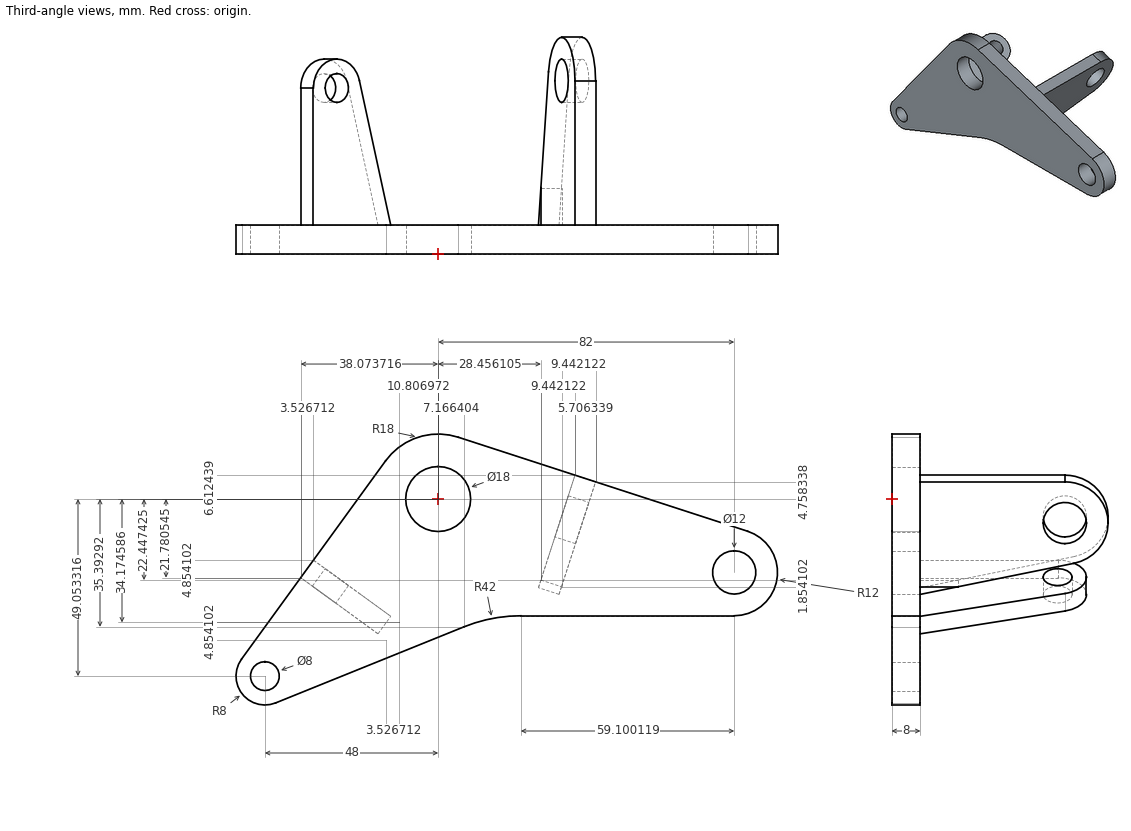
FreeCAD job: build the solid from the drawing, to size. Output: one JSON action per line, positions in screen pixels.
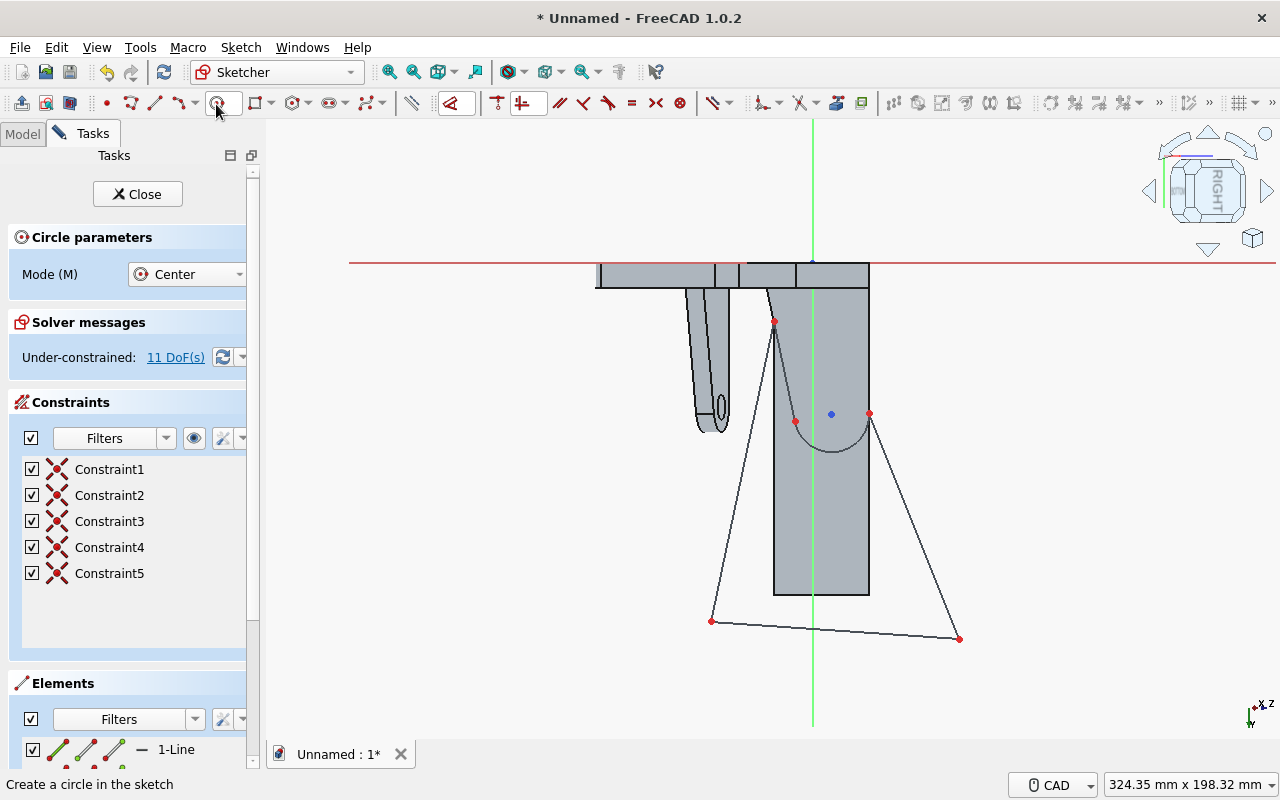
{"action": "left_click", "coordinate": [832, 413]}
{"action": "mouse_move", "coordinate": [845, 400]}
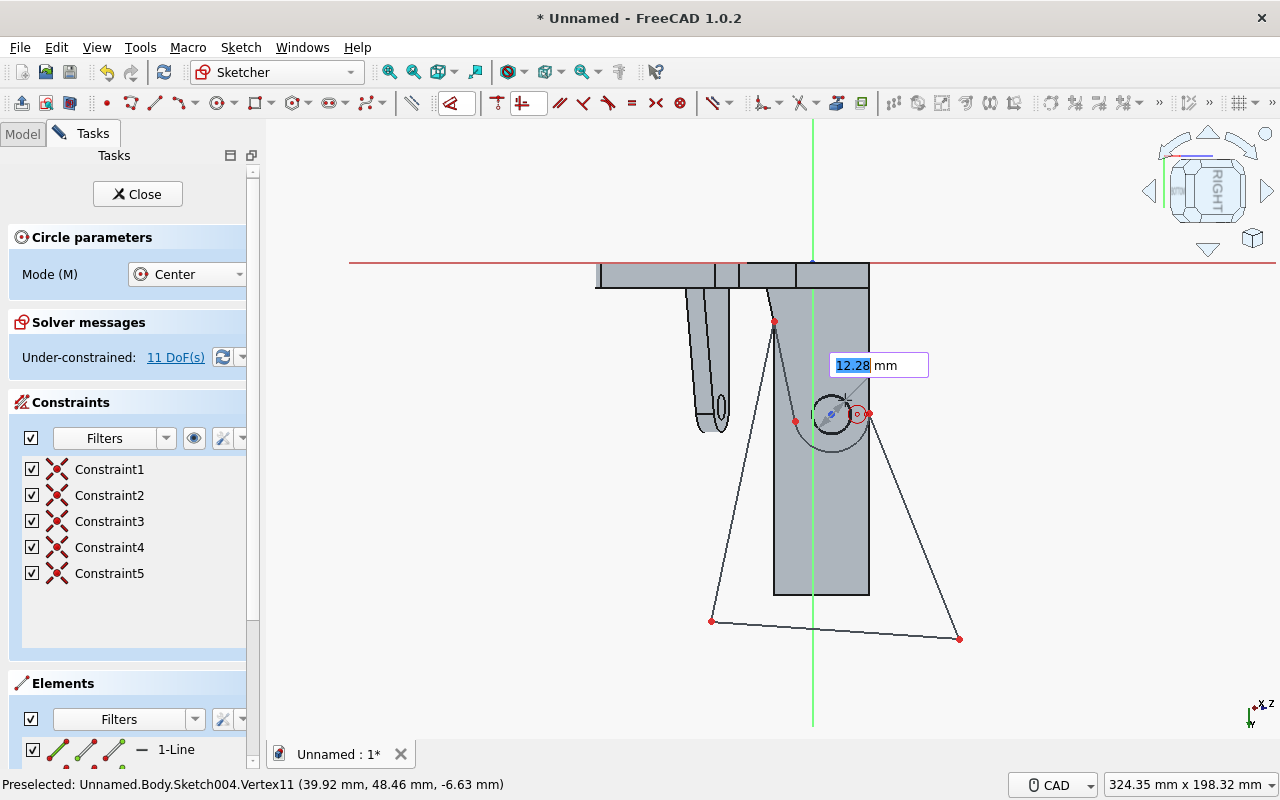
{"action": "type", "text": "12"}
{"action": "key", "text": "Return"}
{"action": "key", "text": "Escape"}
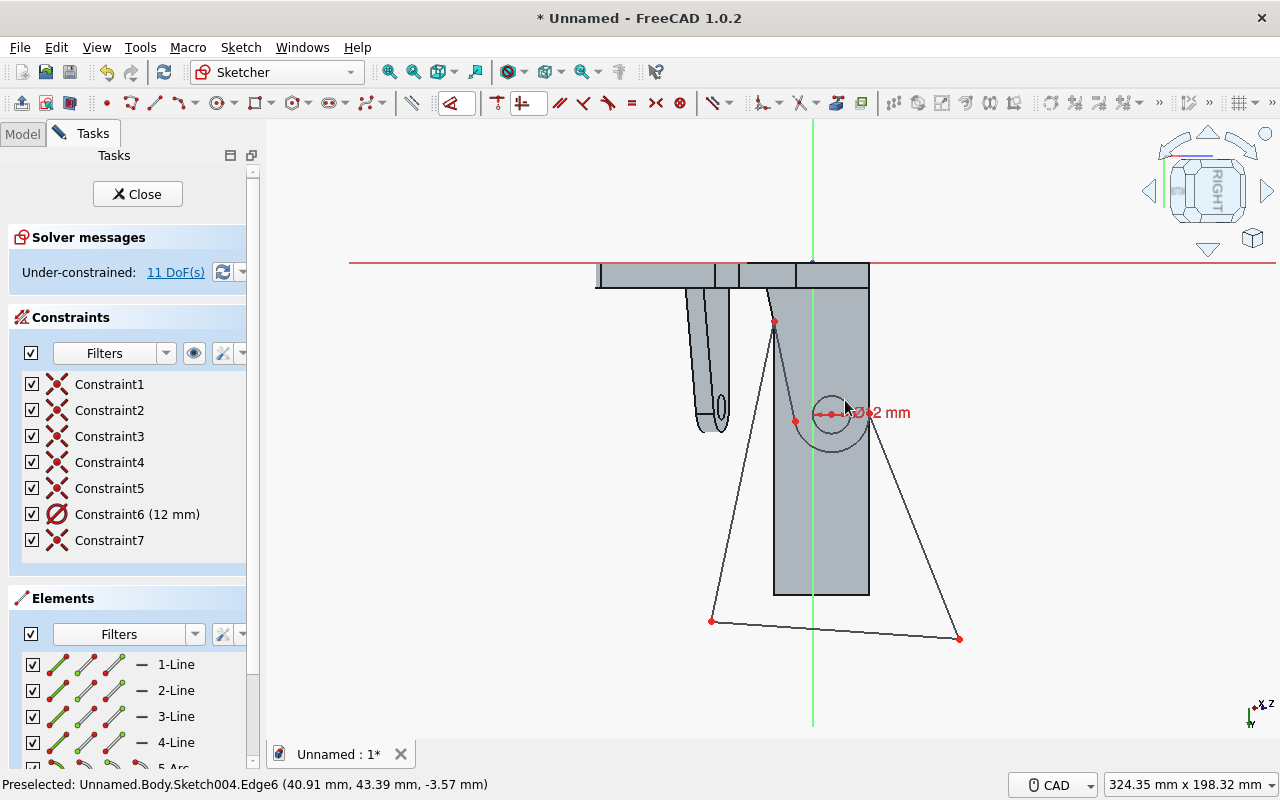
{"action": "left_click", "coordinate": [789, 392]}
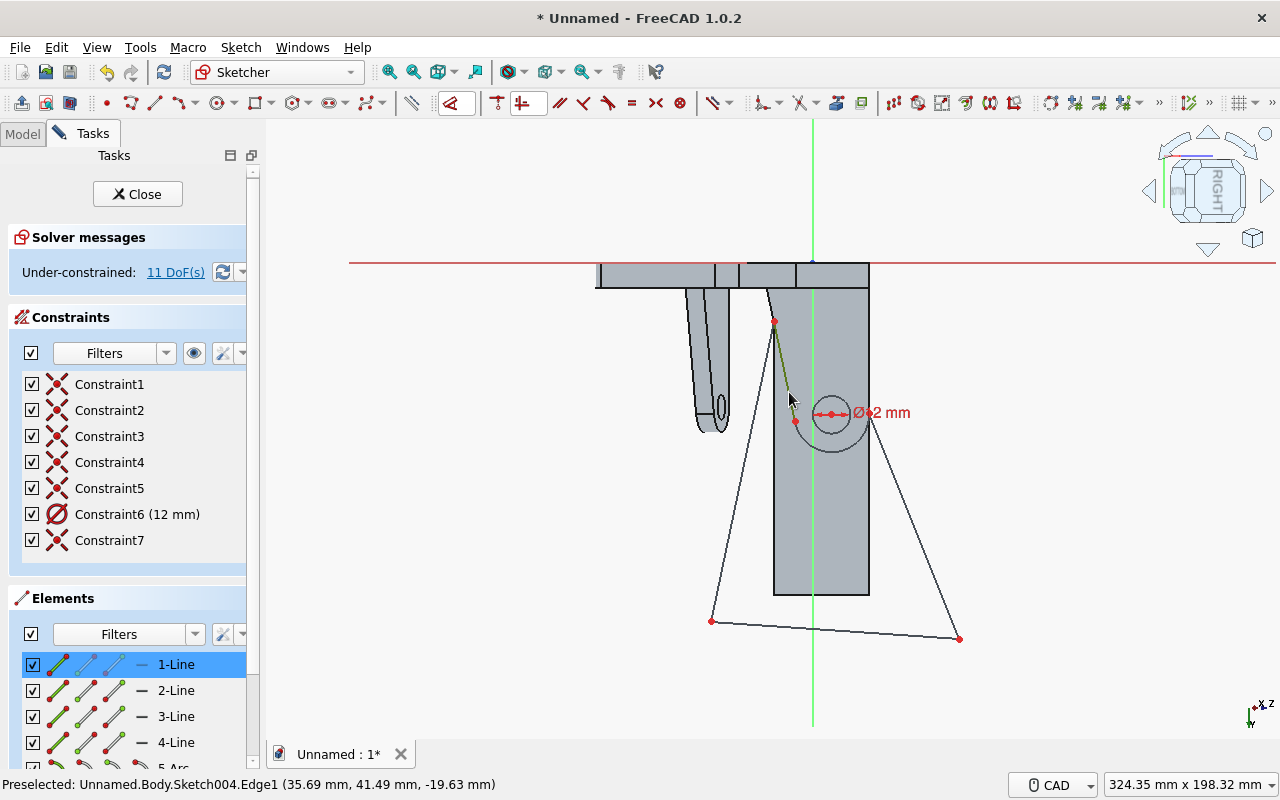
{"action": "left_click", "coordinate": [814, 448]}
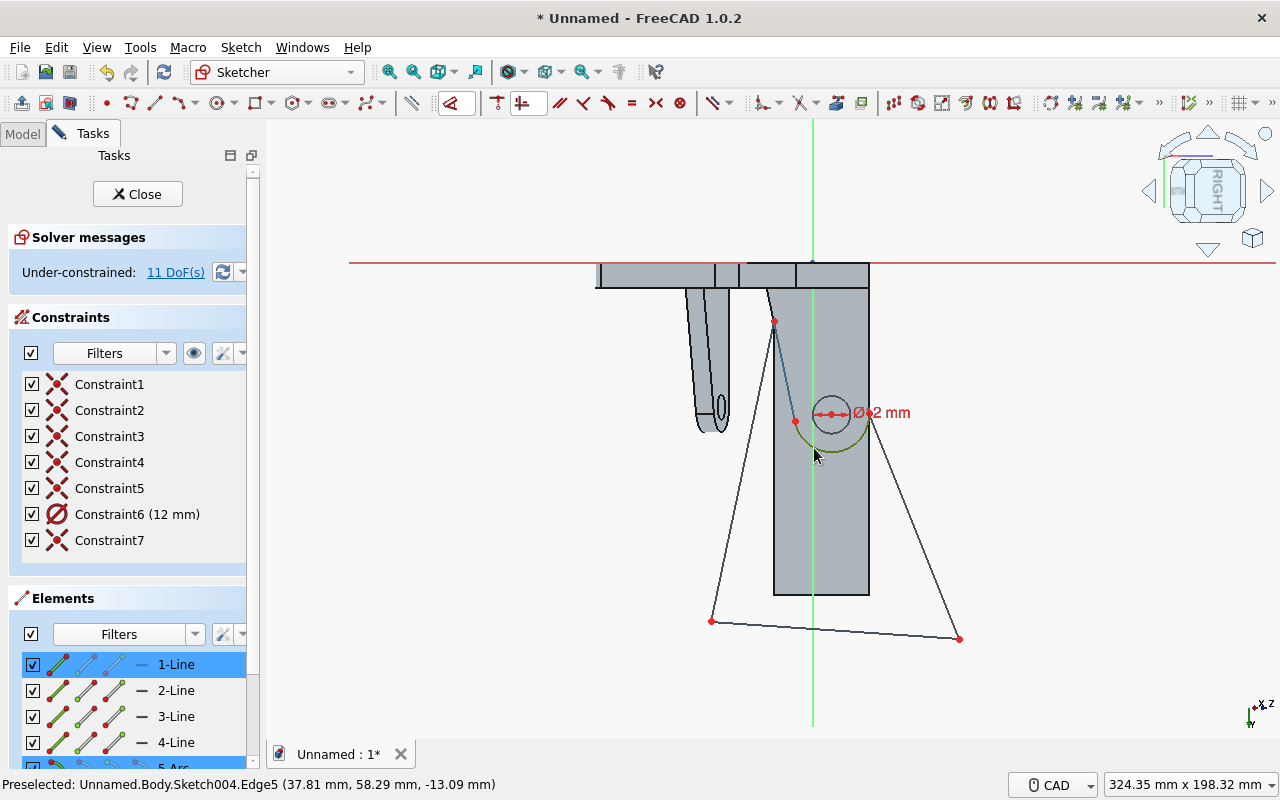
{"action": "key", "text": "t"}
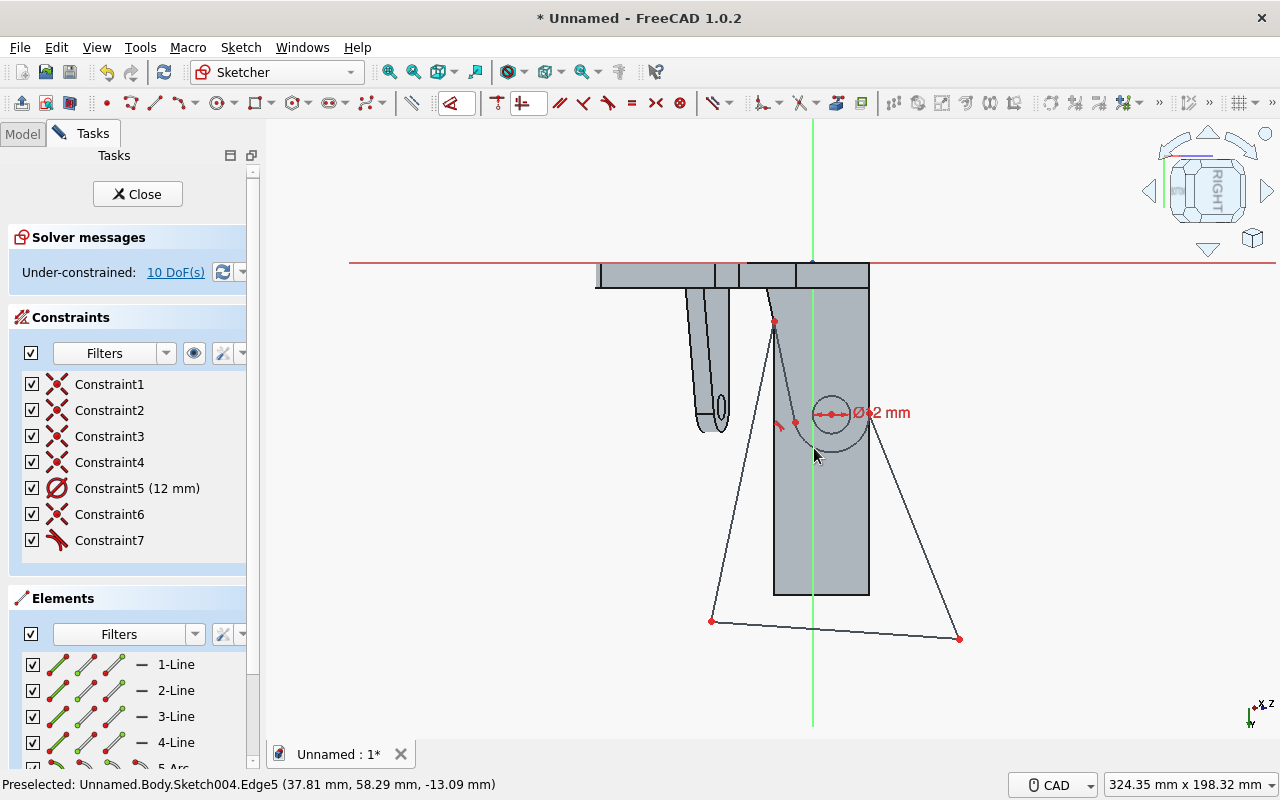
{"action": "left_click", "coordinate": [814, 448]}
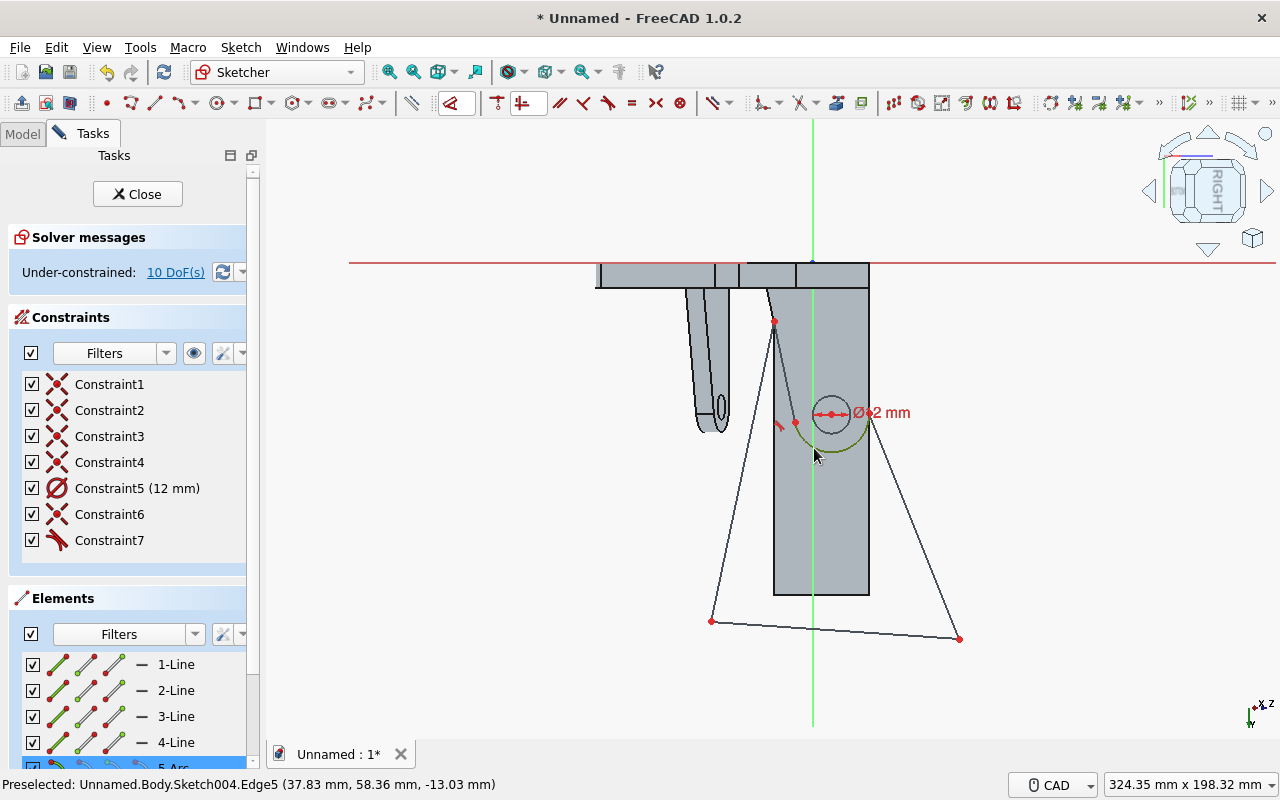
{"action": "left_click", "coordinate": [470, 104]}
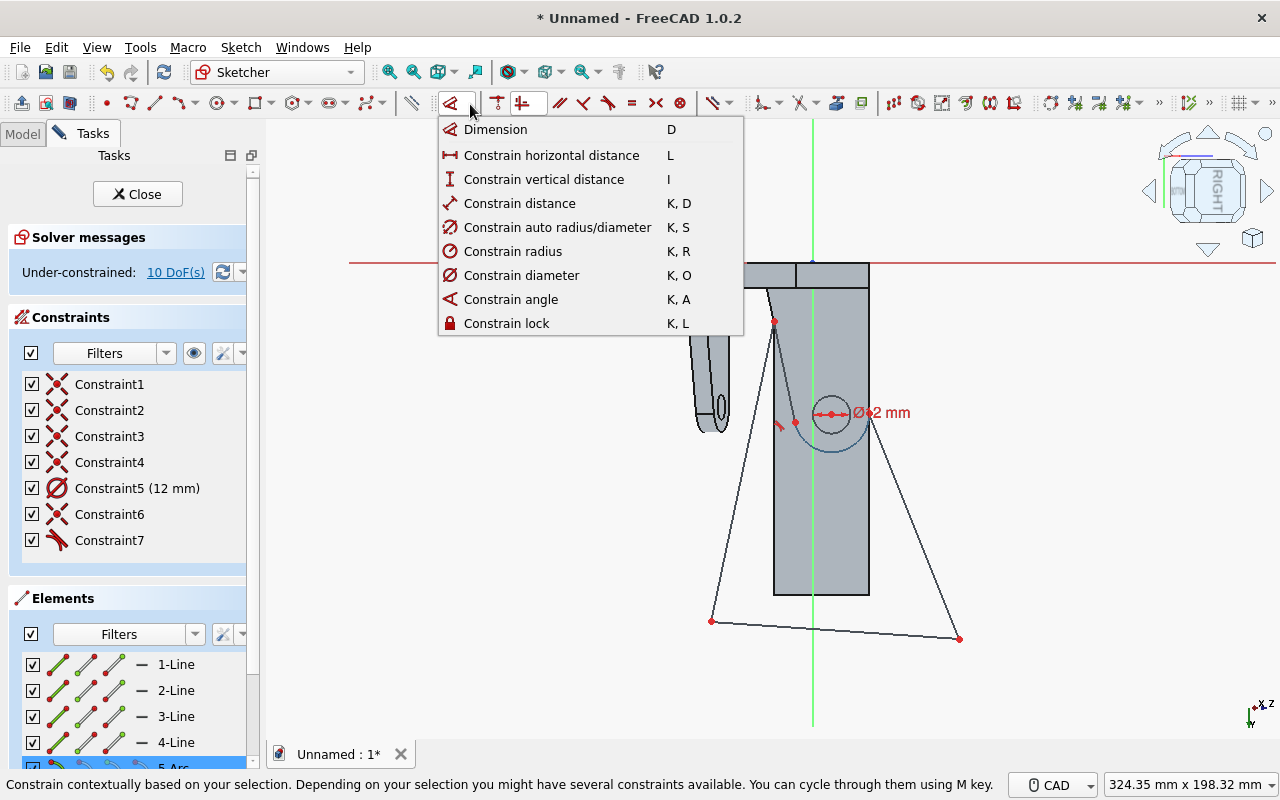
{"action": "left_click", "coordinate": [591, 251]}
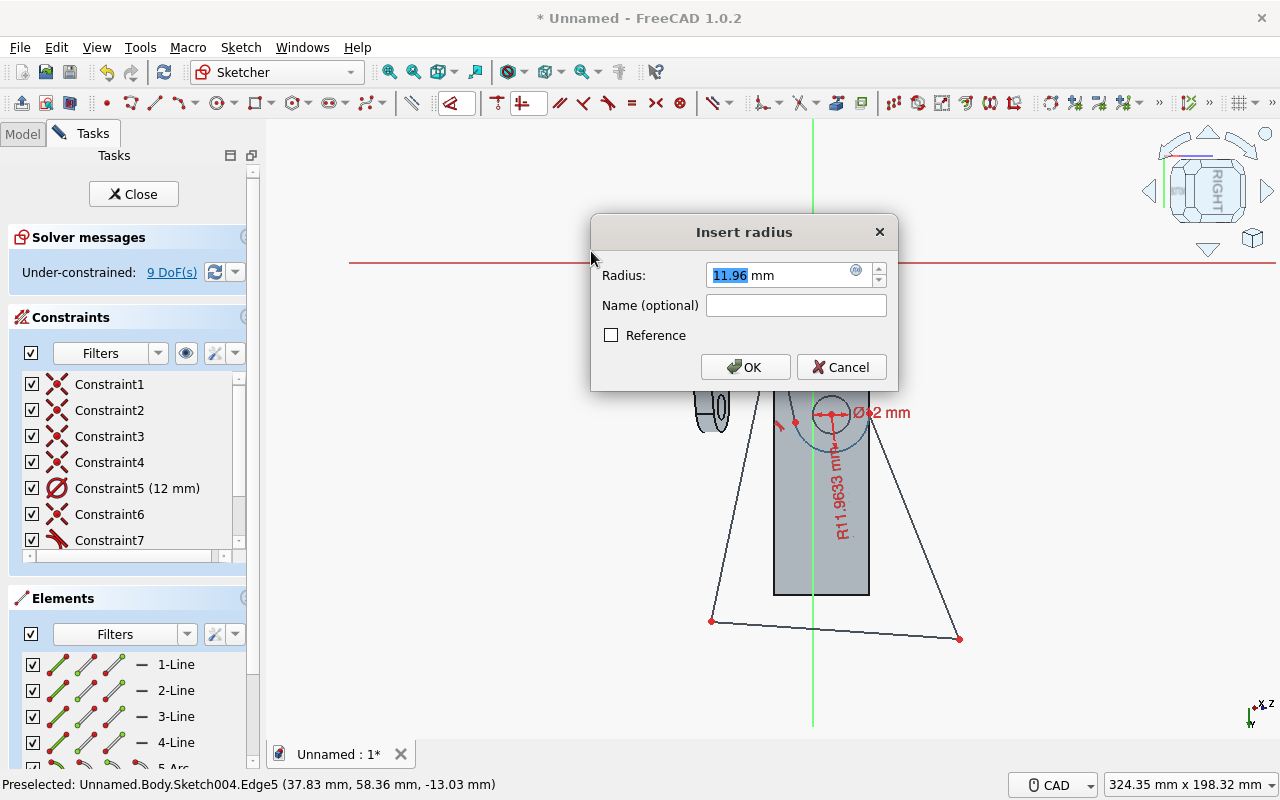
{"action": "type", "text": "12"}
{"action": "key", "text": "Return"}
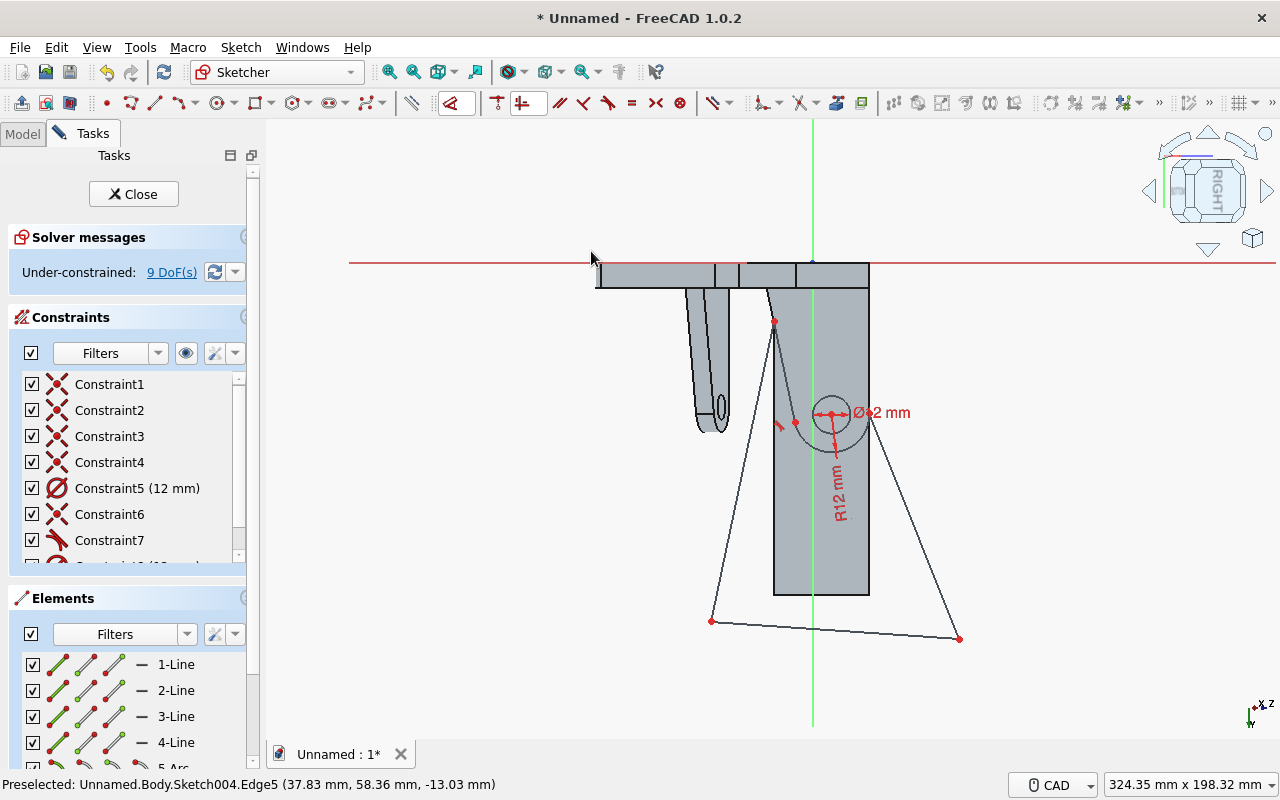
{"action": "left_click", "coordinate": [832, 415]}